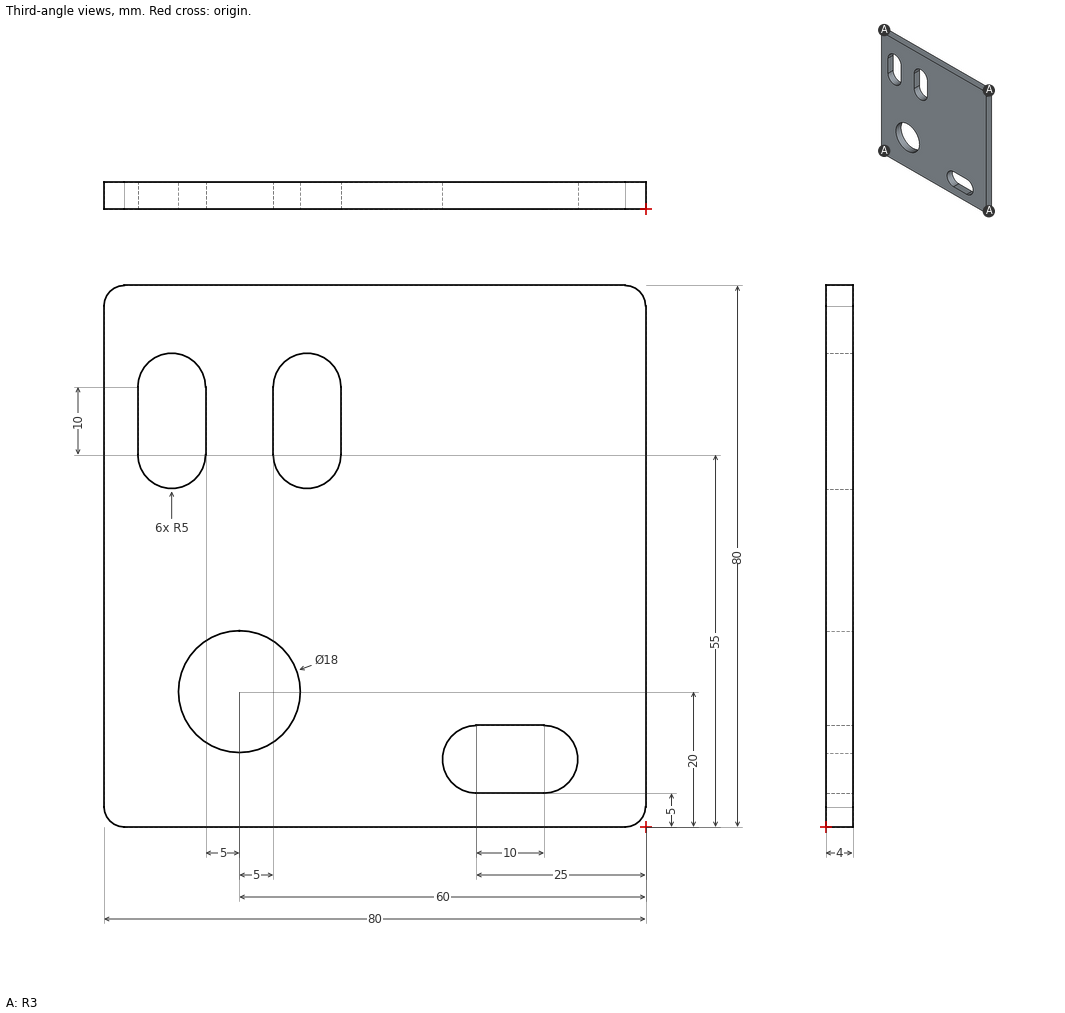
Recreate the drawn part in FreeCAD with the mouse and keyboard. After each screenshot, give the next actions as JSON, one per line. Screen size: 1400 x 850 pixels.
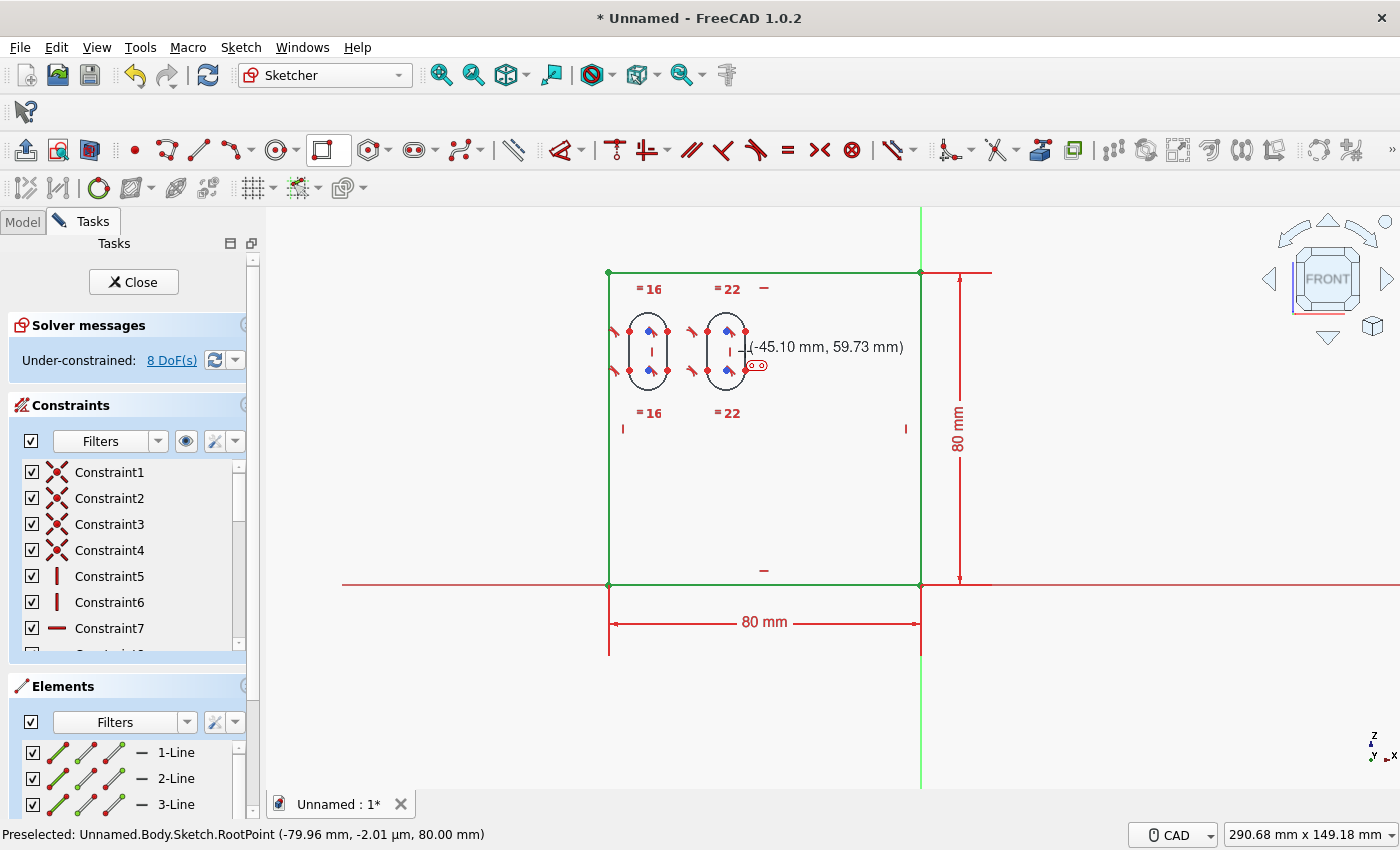
{"action": "left_click", "coordinate": [823, 546]}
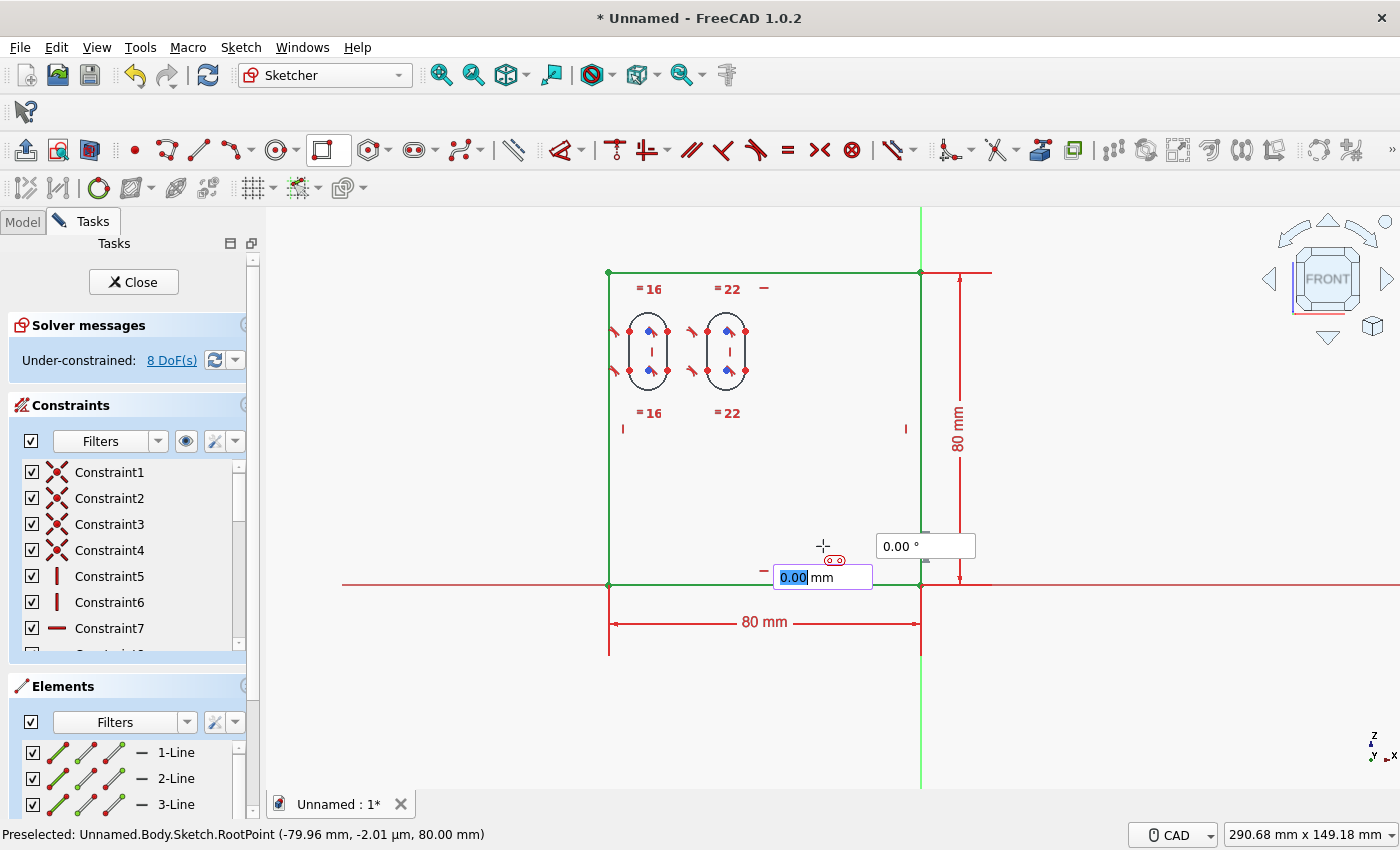
{"action": "left_click", "coordinate": [862, 546]}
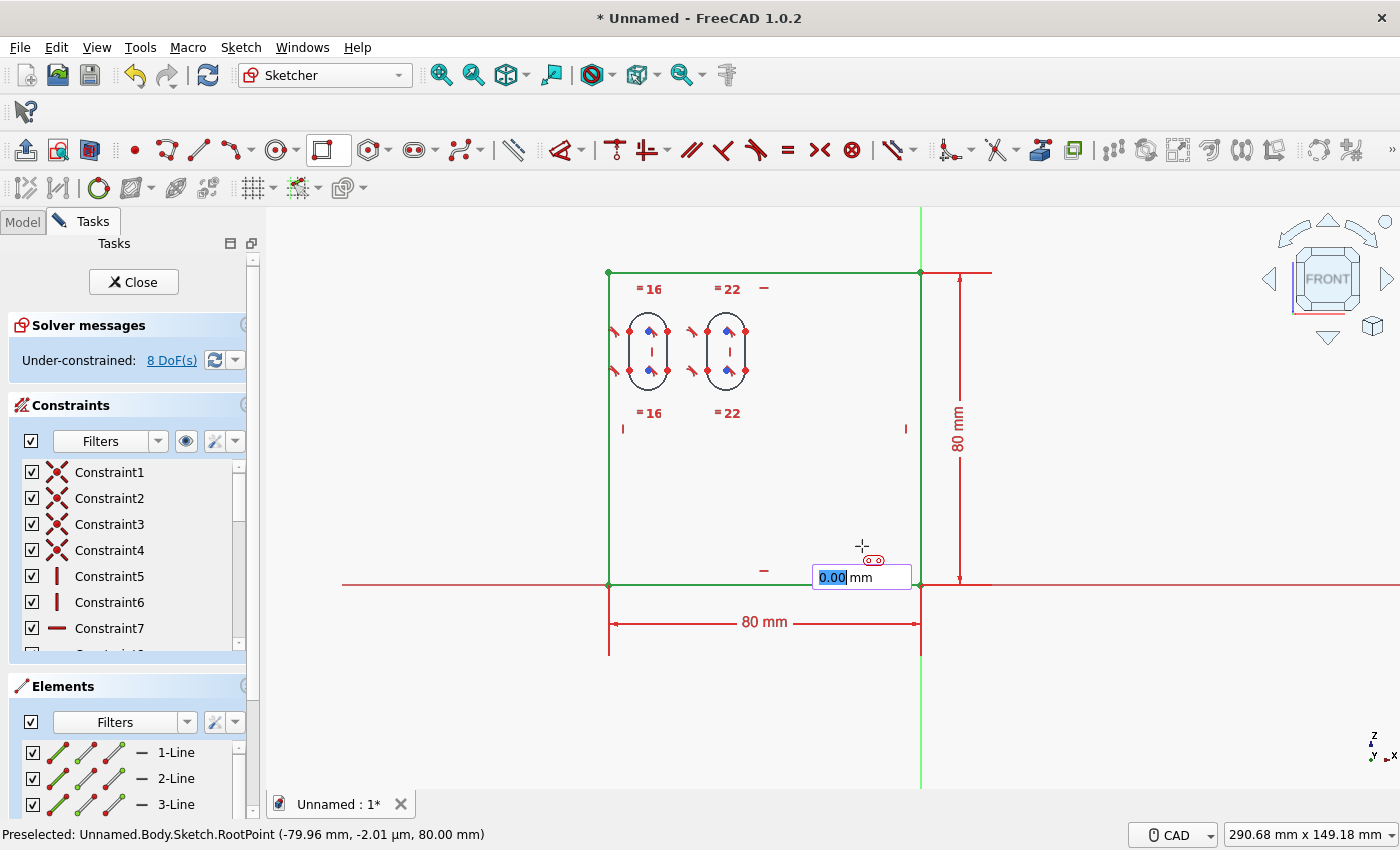
{"action": "left_click", "coordinate": [843, 566]}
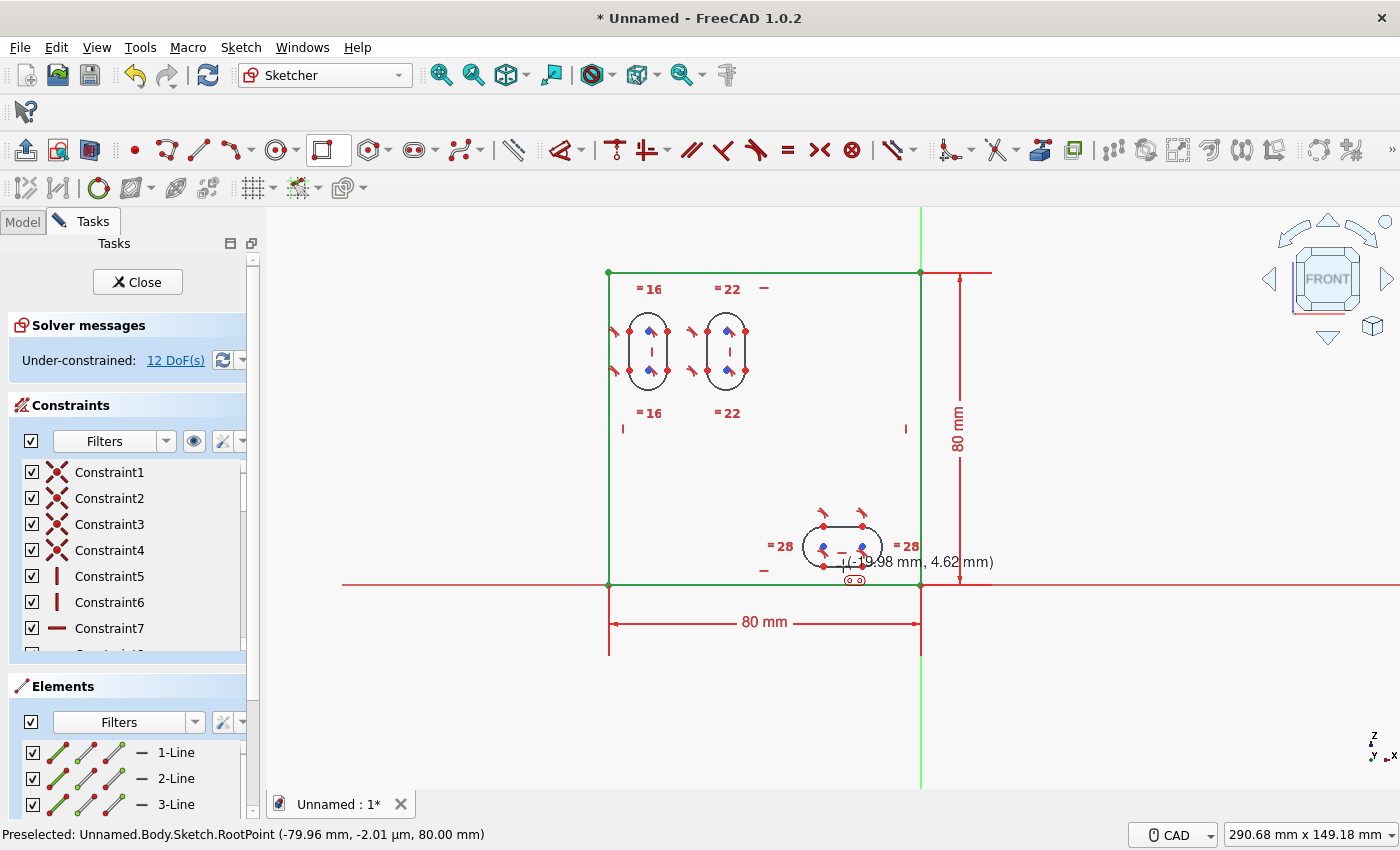
{"action": "left_click", "coordinate": [276, 150]}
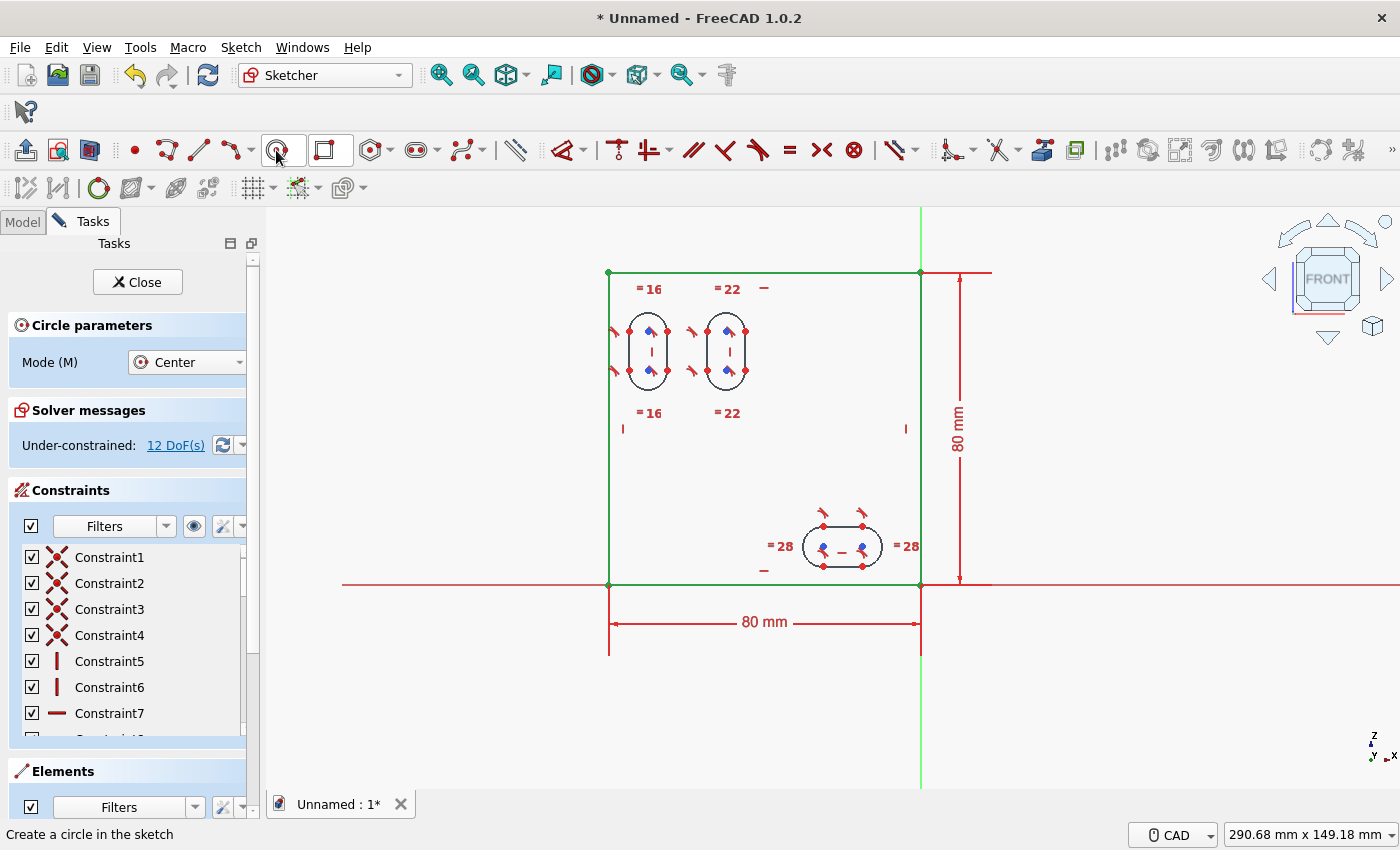
{"action": "left_click", "coordinate": [687, 507]}
{"action": "mouse_move", "coordinate": [712, 482]}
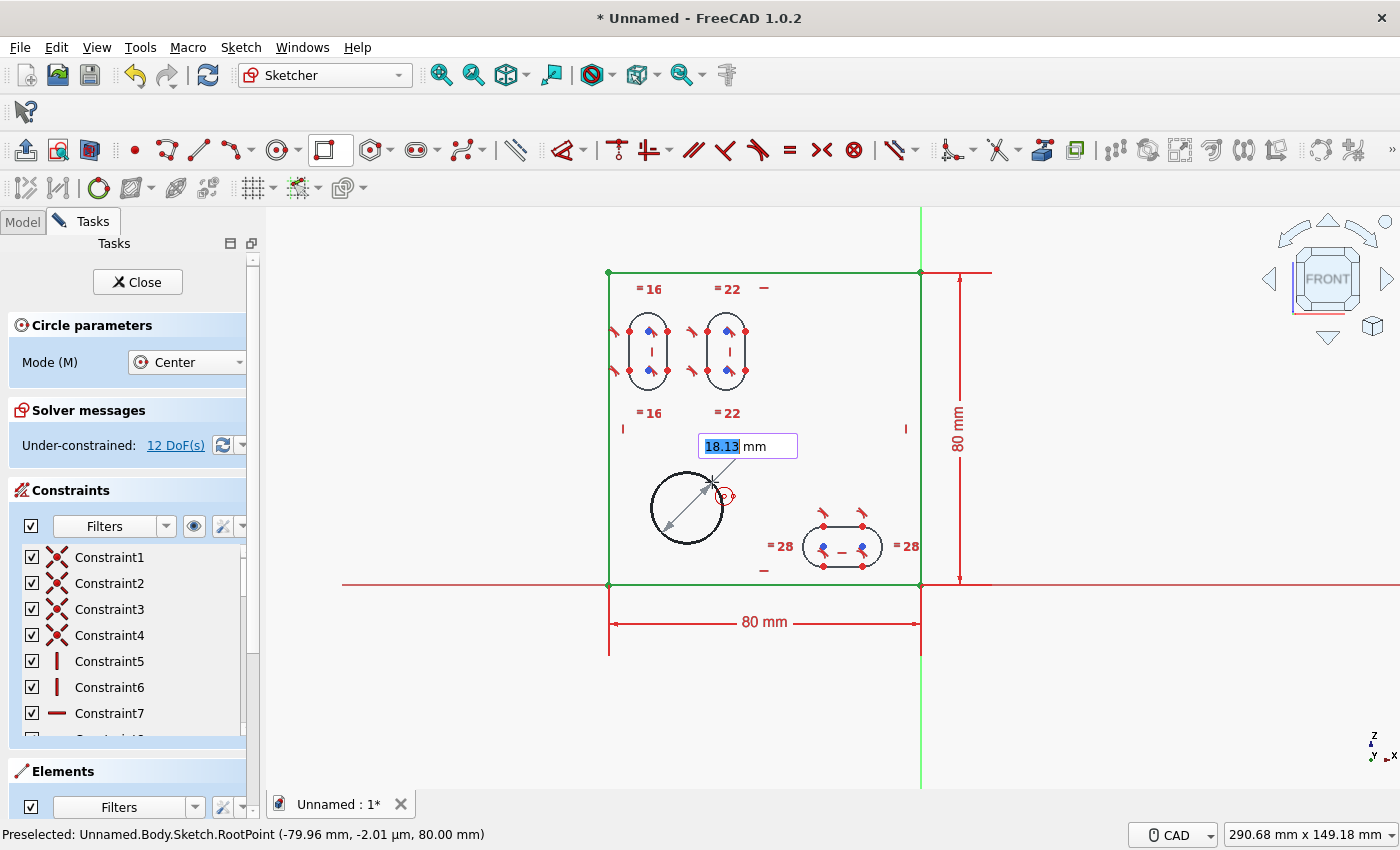
{"action": "type", "text": "18"}
{"action": "key", "text": "Return"}
{"action": "key", "text": "Escape"}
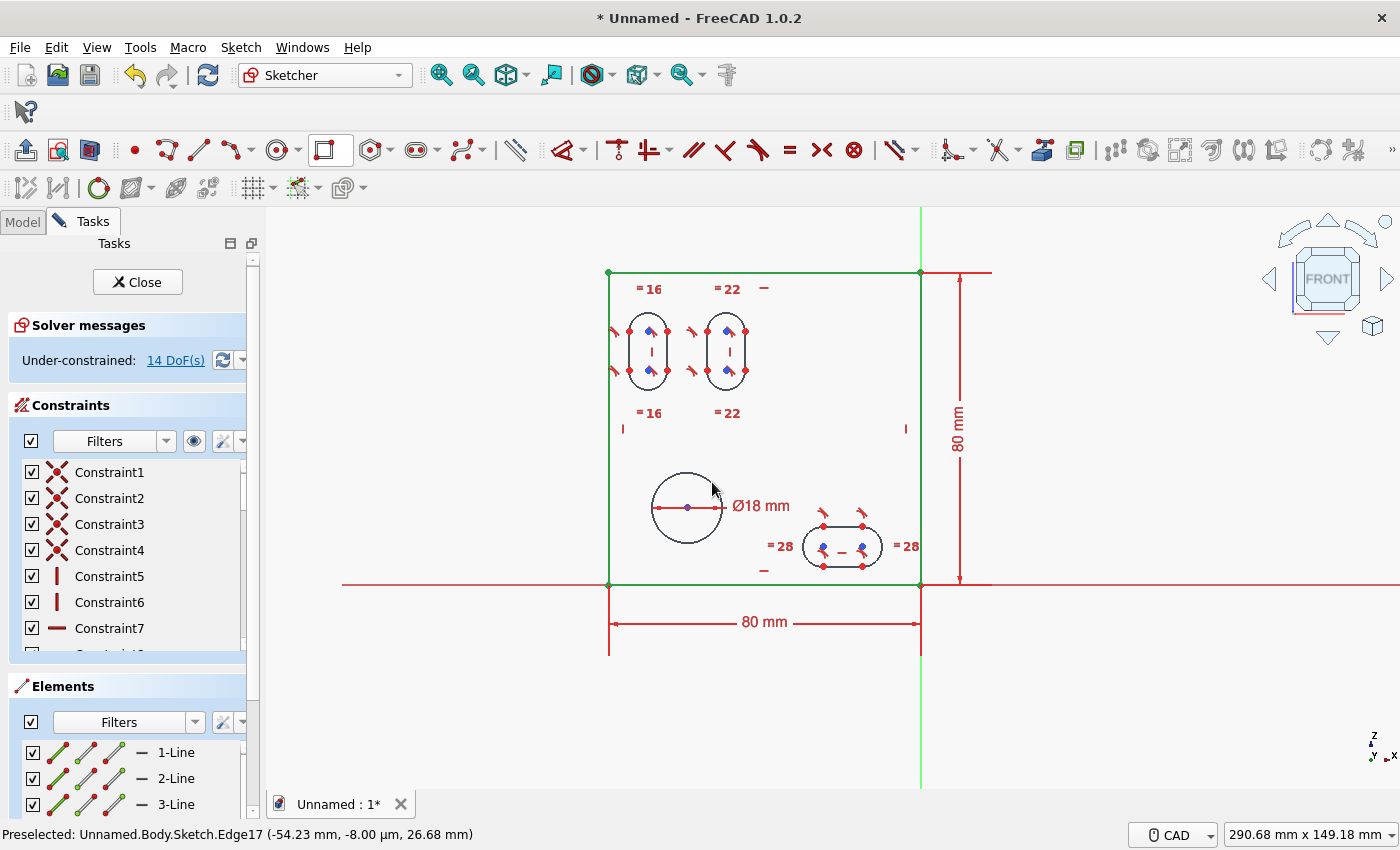
{"action": "left_click", "coordinate": [637, 386]}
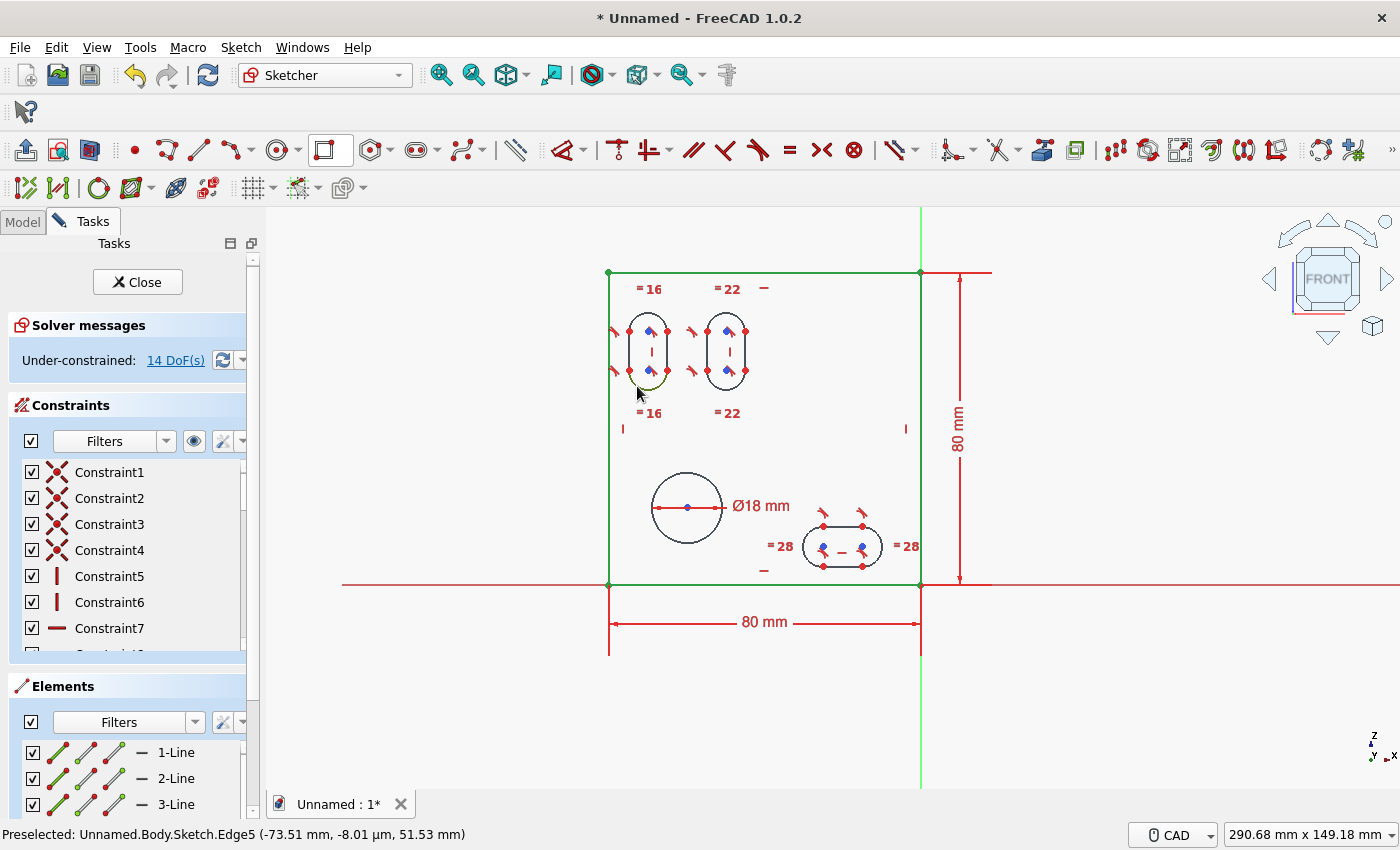
{"action": "left_click", "coordinate": [715, 386]}